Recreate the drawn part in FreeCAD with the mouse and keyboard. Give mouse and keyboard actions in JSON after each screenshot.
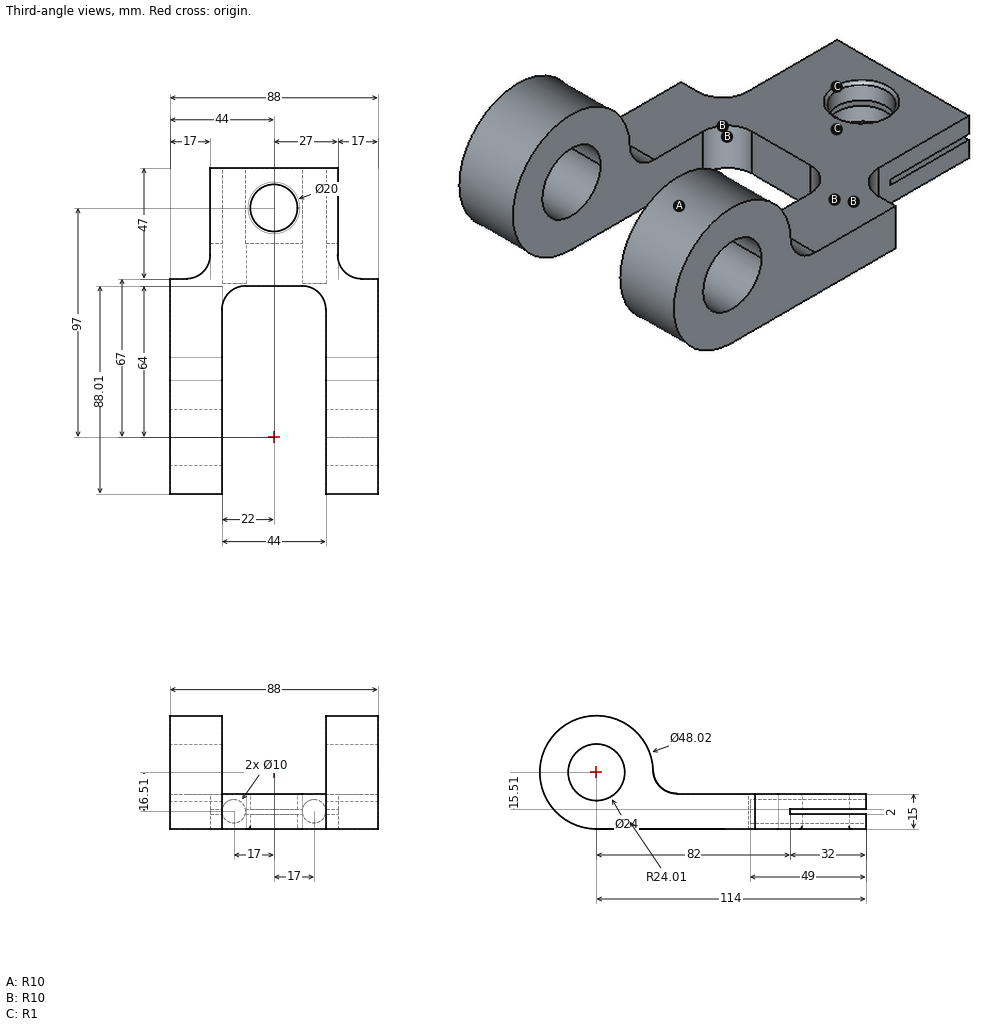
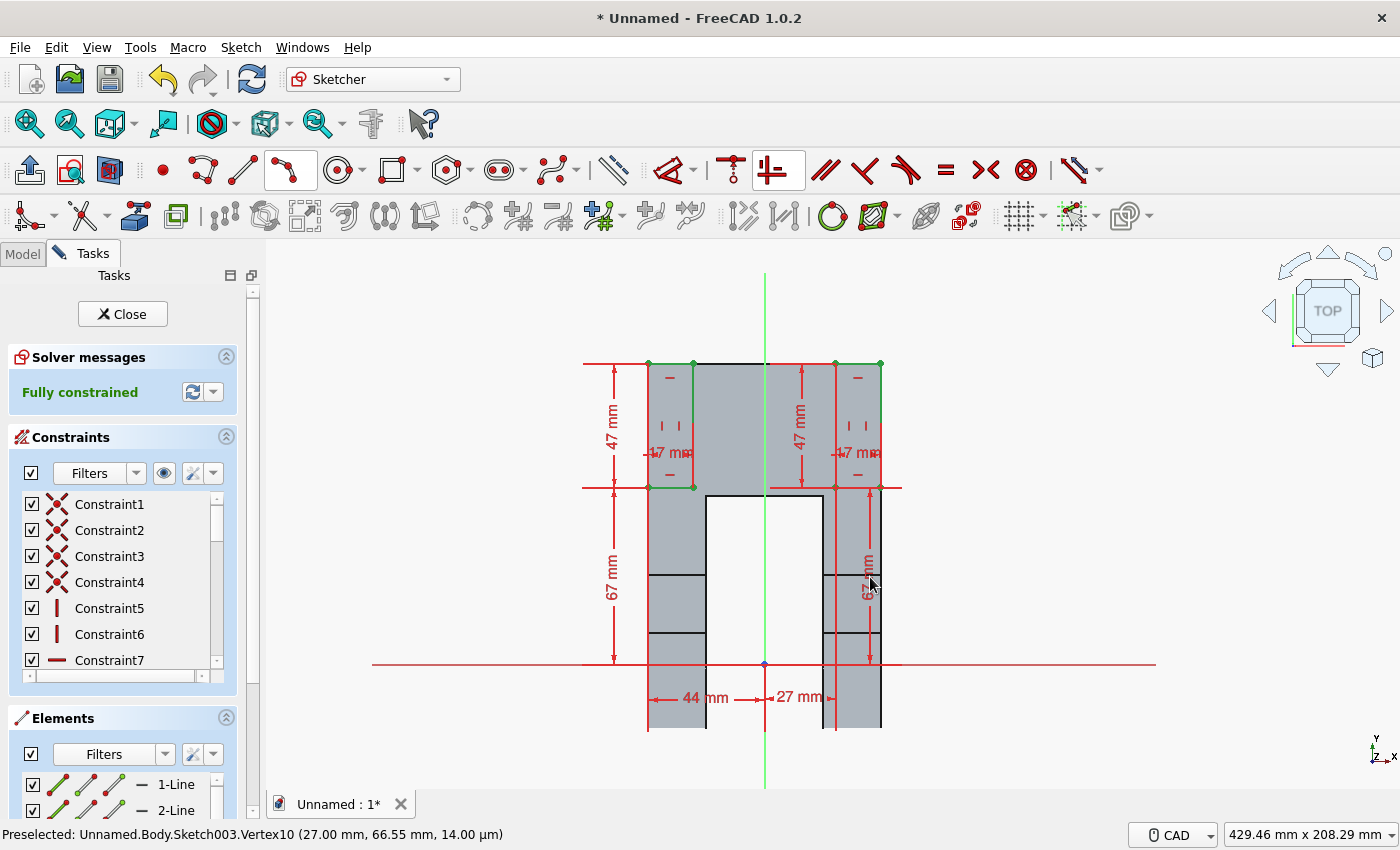
{"action": "left_click", "coordinate": [123, 314]}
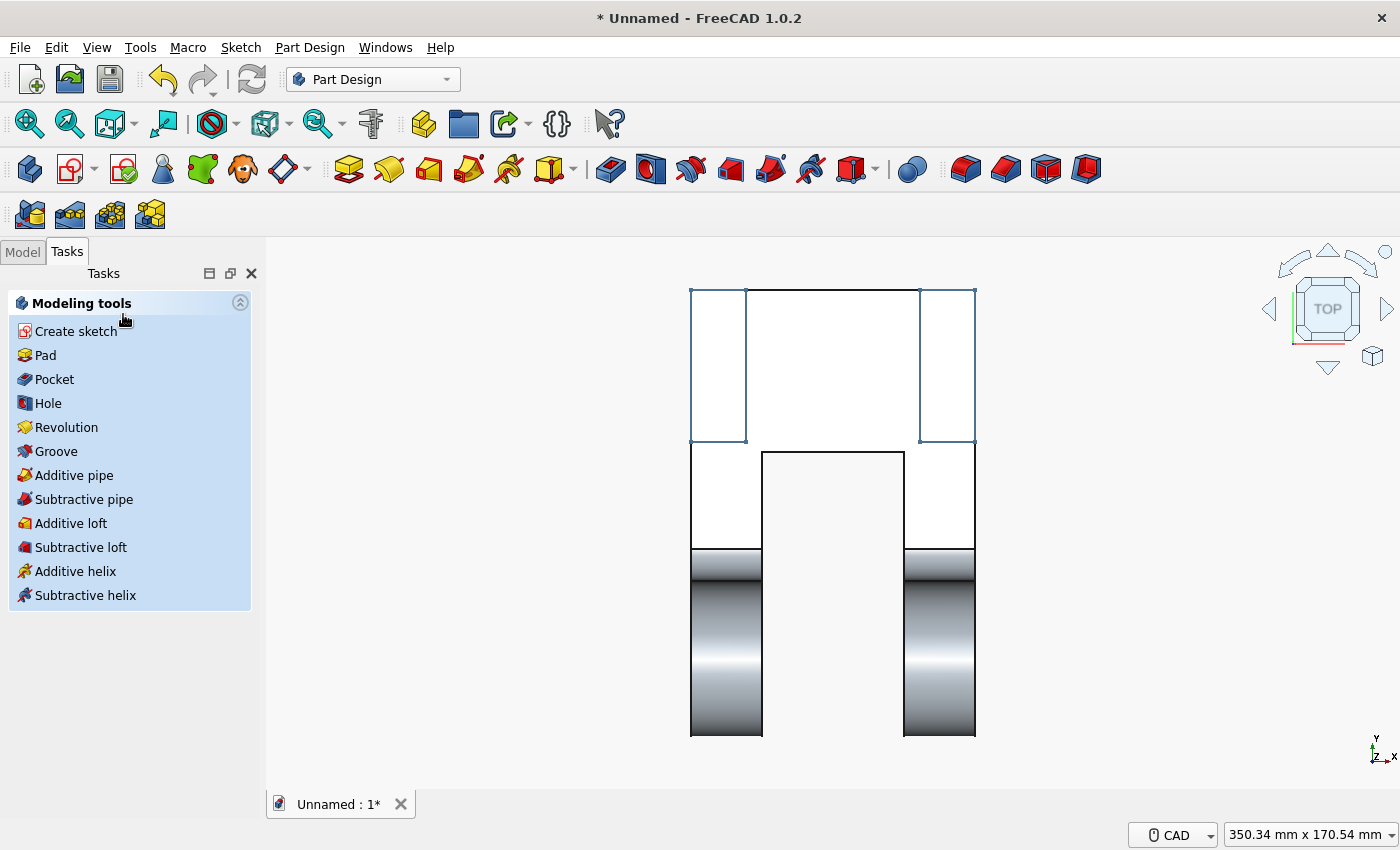
{"action": "left_click", "coordinate": [612, 170]}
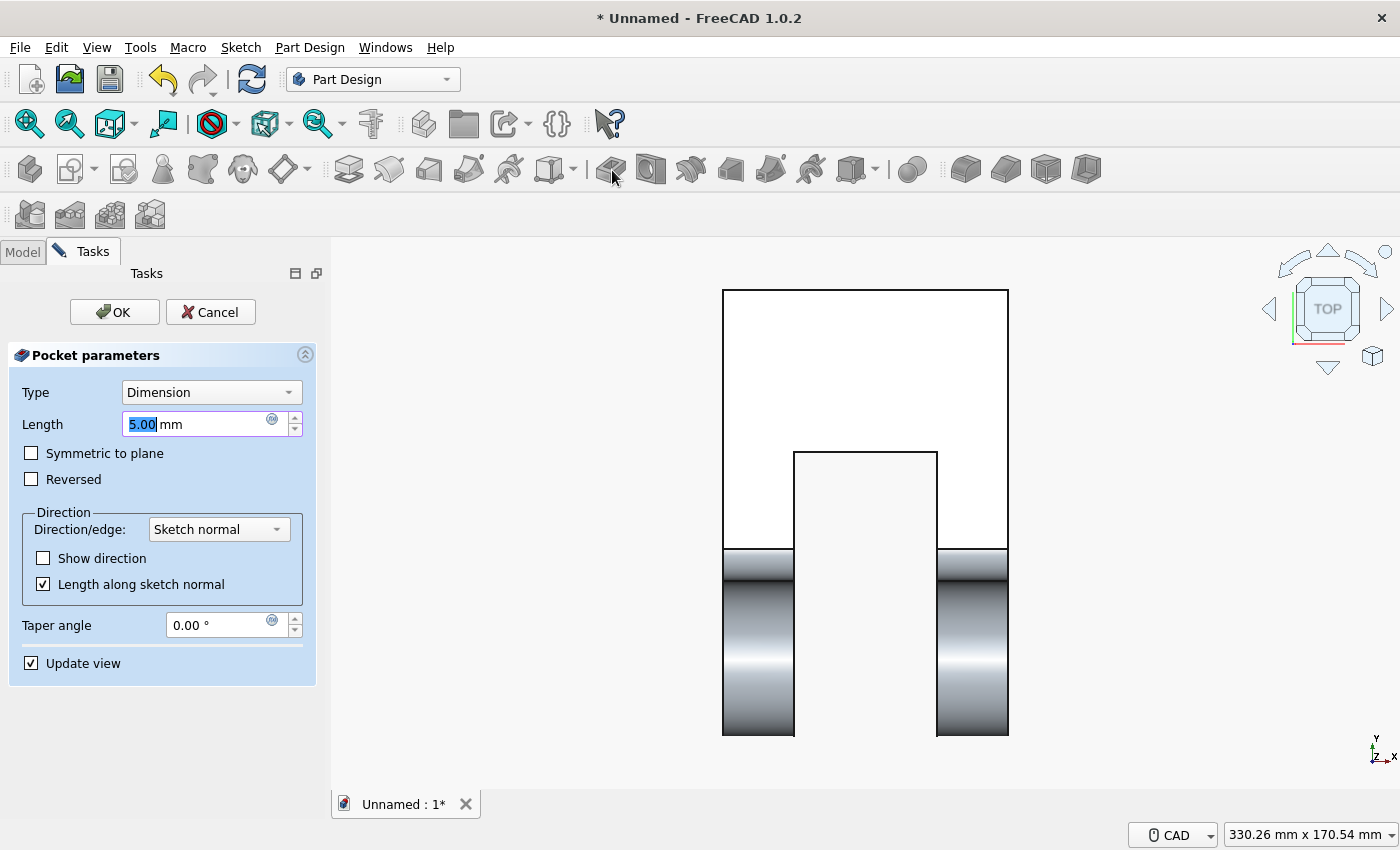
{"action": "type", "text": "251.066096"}
{"action": "key", "text": "Tab"}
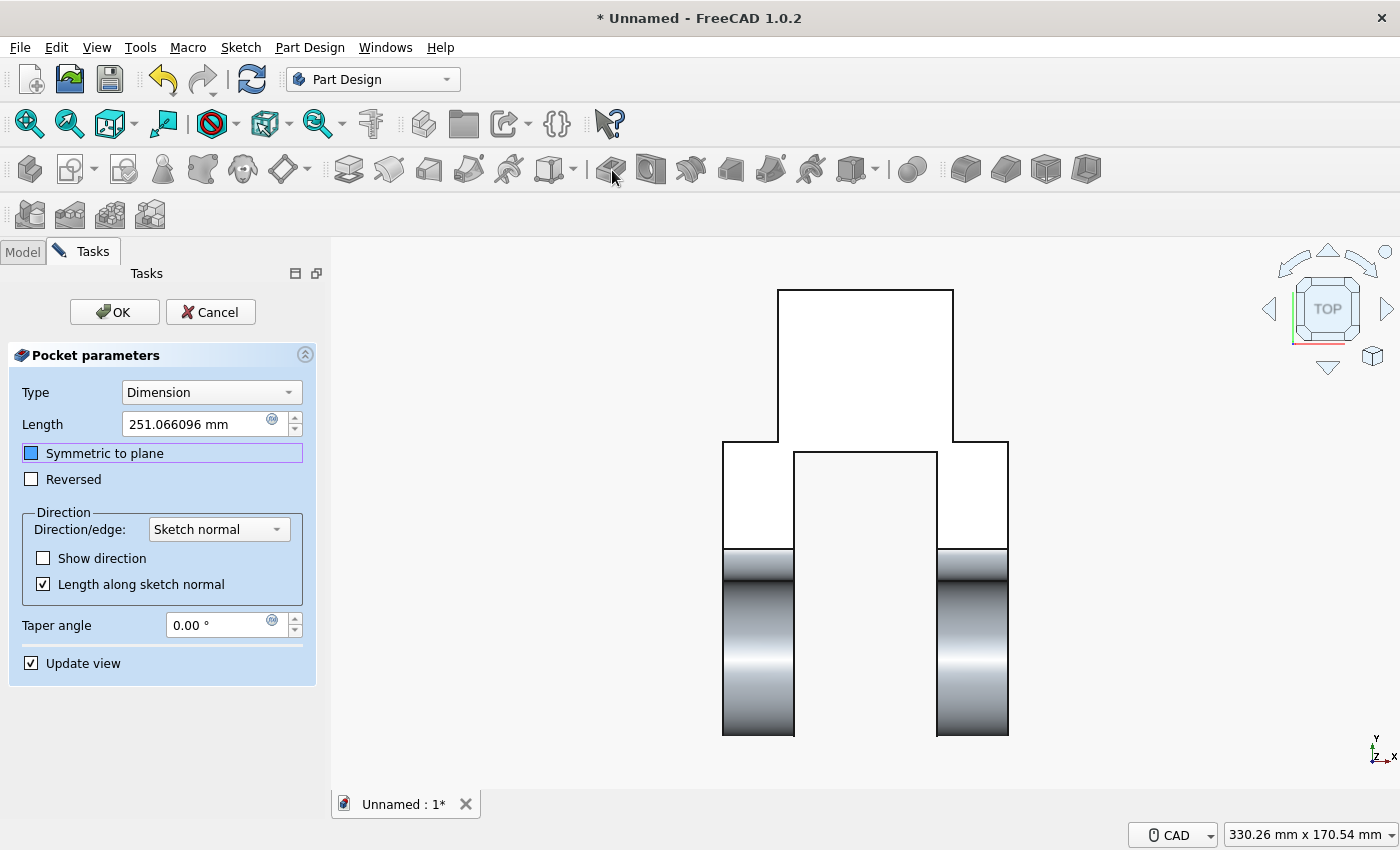
{"action": "left_click", "coordinate": [30, 453]}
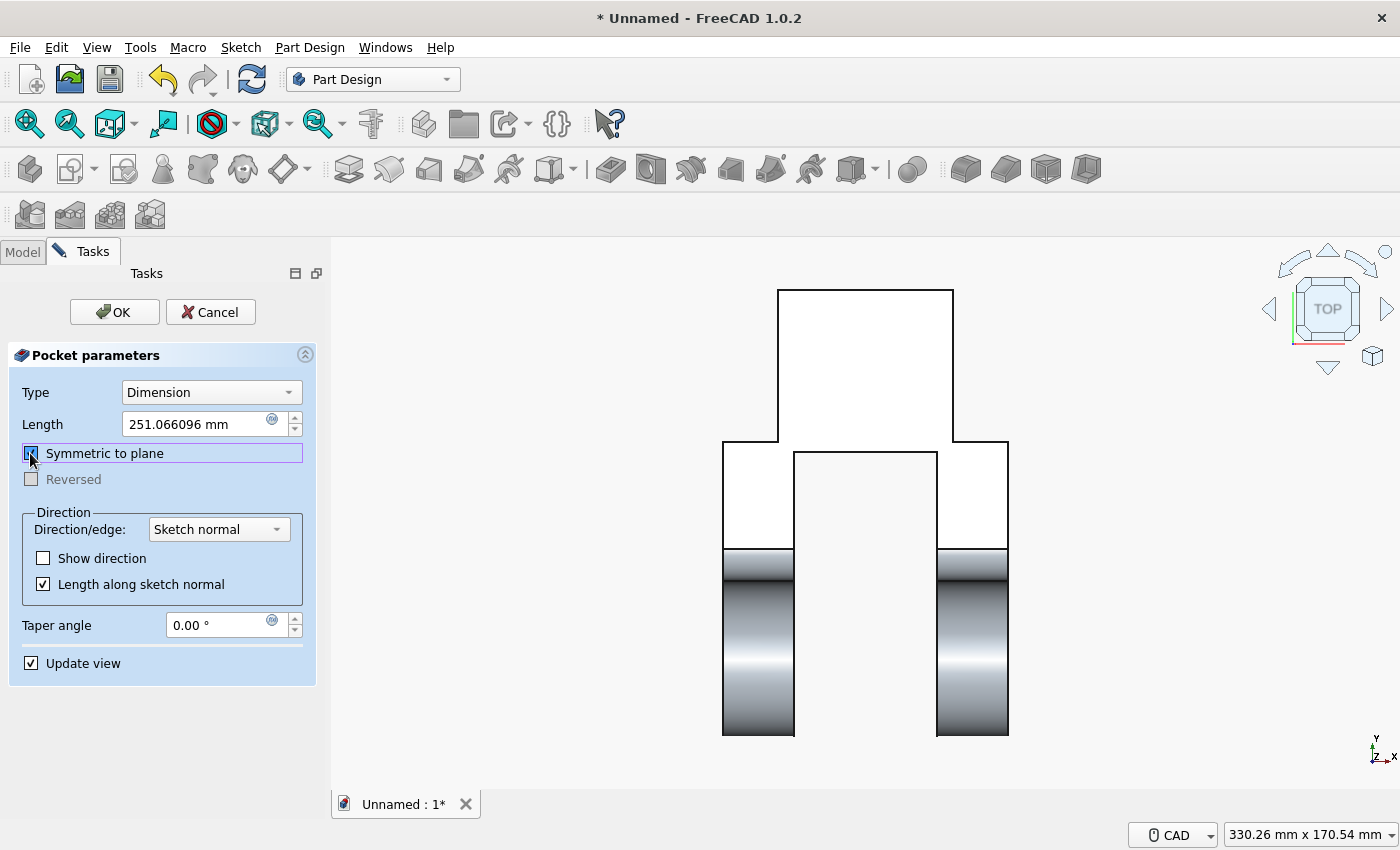
{"action": "left_click", "coordinate": [115, 312]}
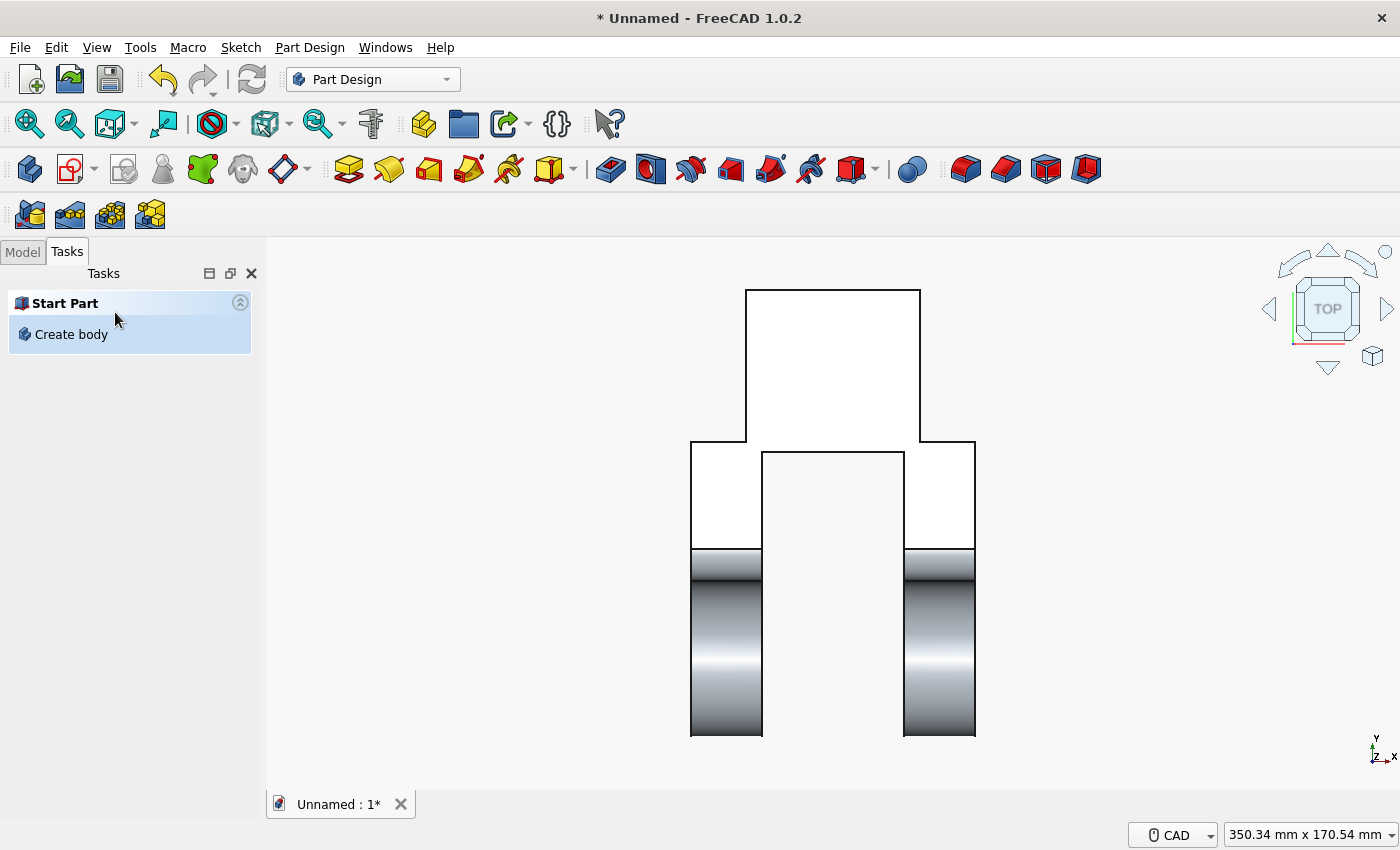
{"action": "key", "text": "0"}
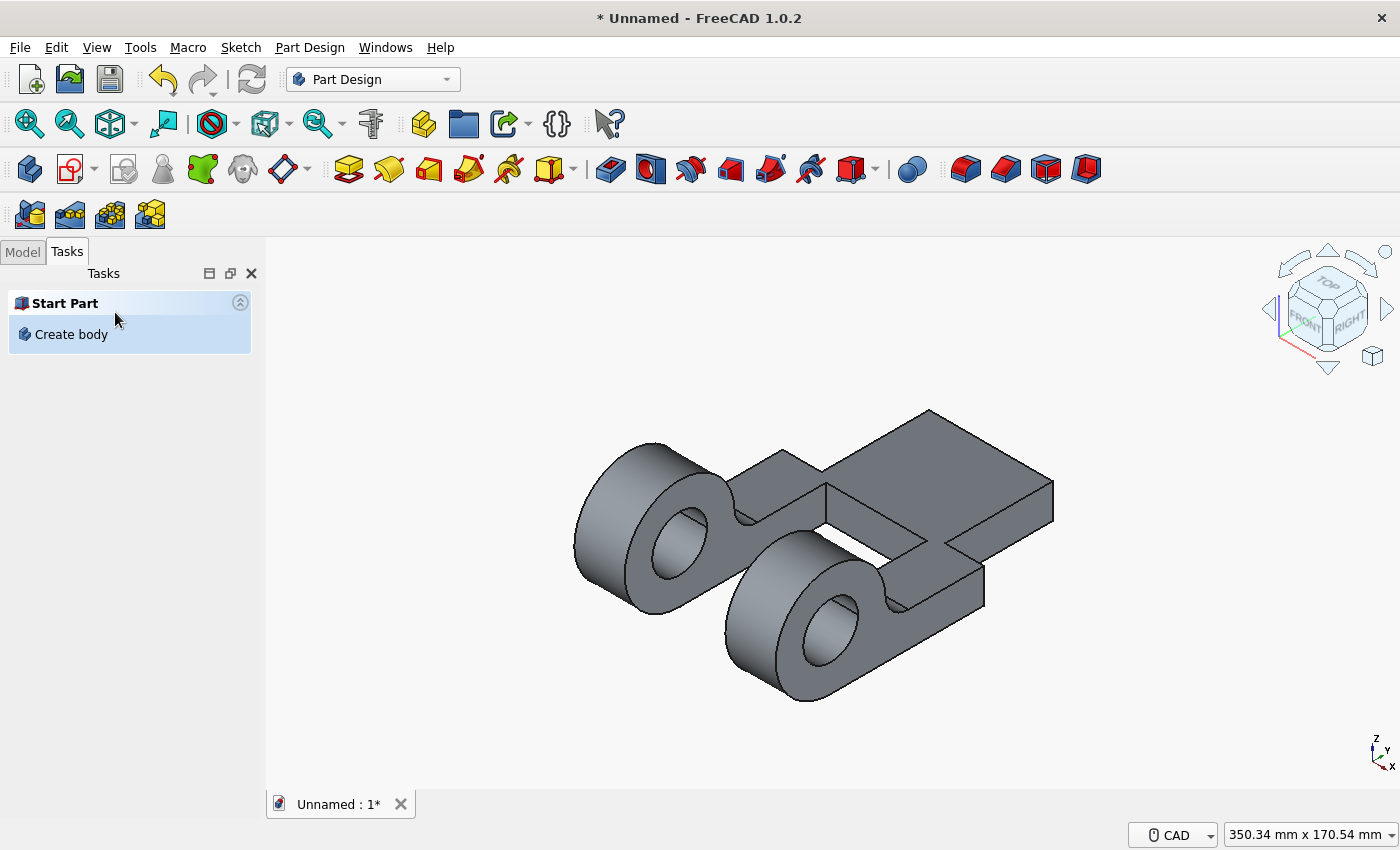
{"action": "key", "text": "2"}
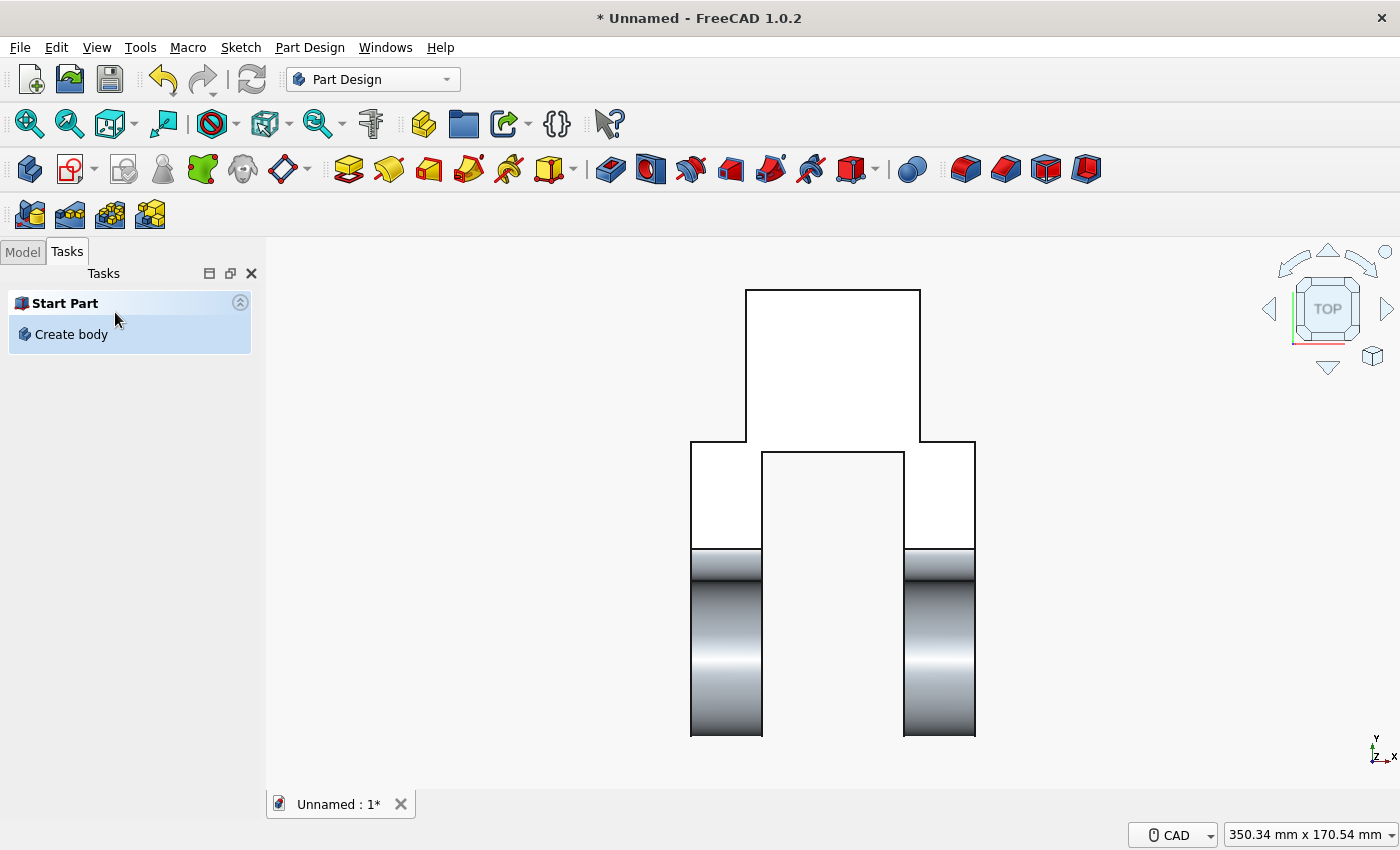
{"action": "key", "text": "1"}